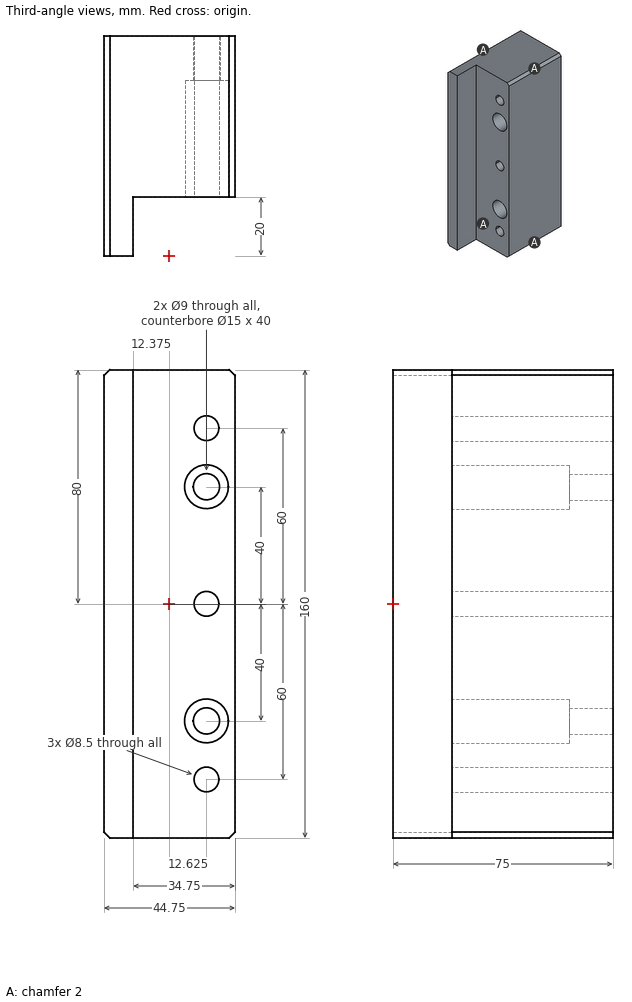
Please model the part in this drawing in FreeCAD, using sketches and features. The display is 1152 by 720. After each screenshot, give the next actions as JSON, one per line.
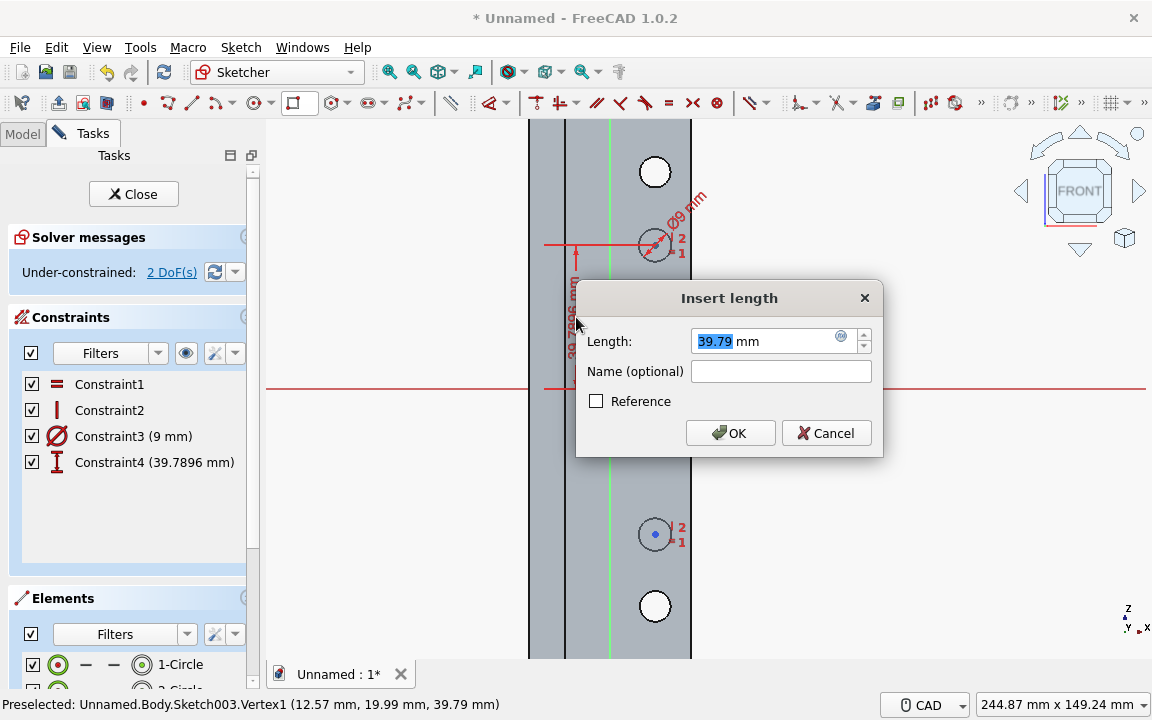
{"action": "type", "text": "40"}
{"action": "key", "text": "Return"}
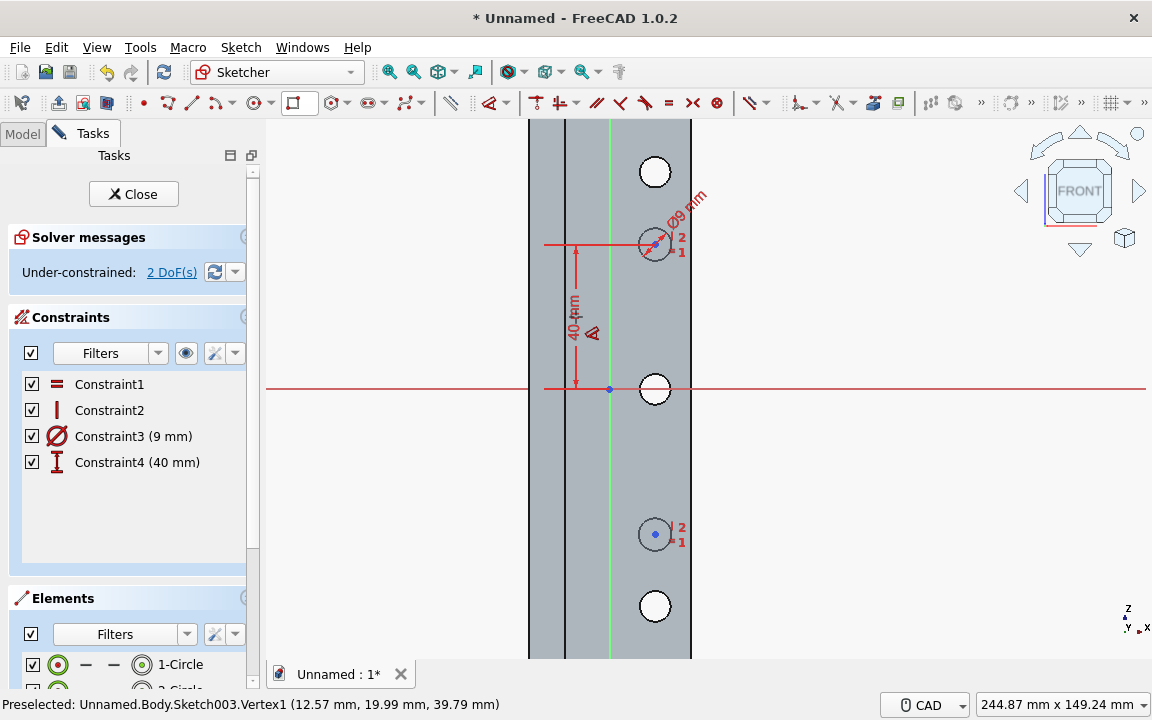
{"action": "left_click", "coordinate": [655, 535]}
{"action": "left_click", "coordinate": [576, 462]}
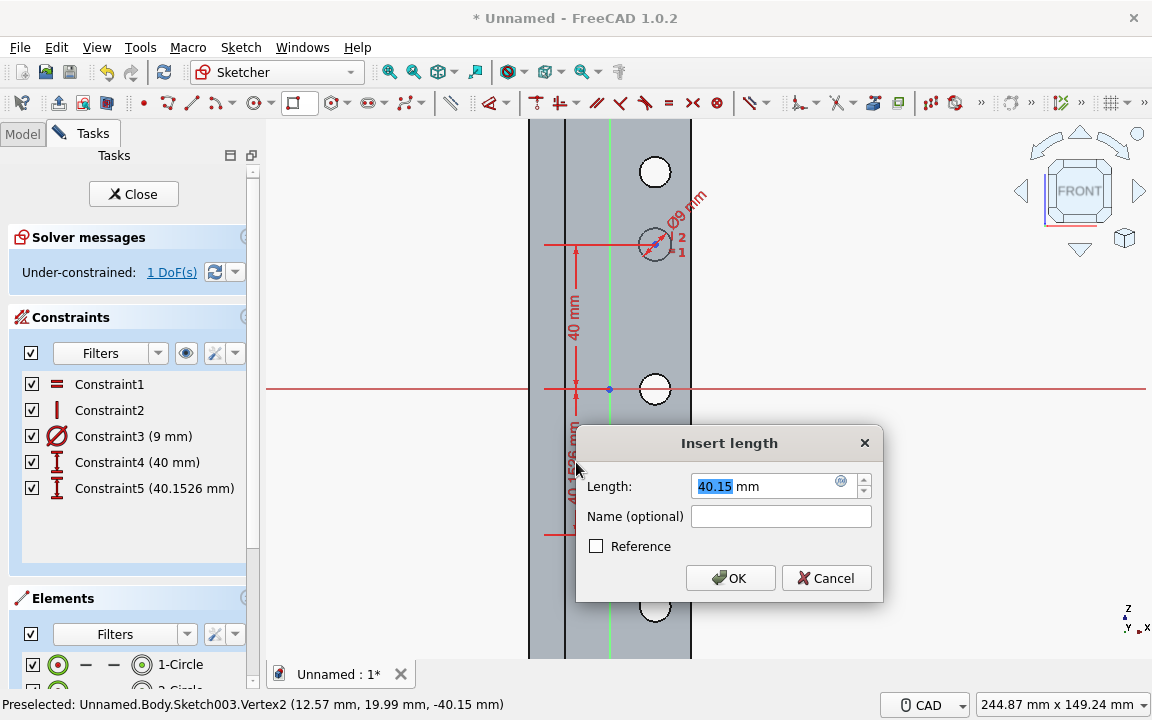
{"action": "type", "text": "40"}
{"action": "key", "text": "Return"}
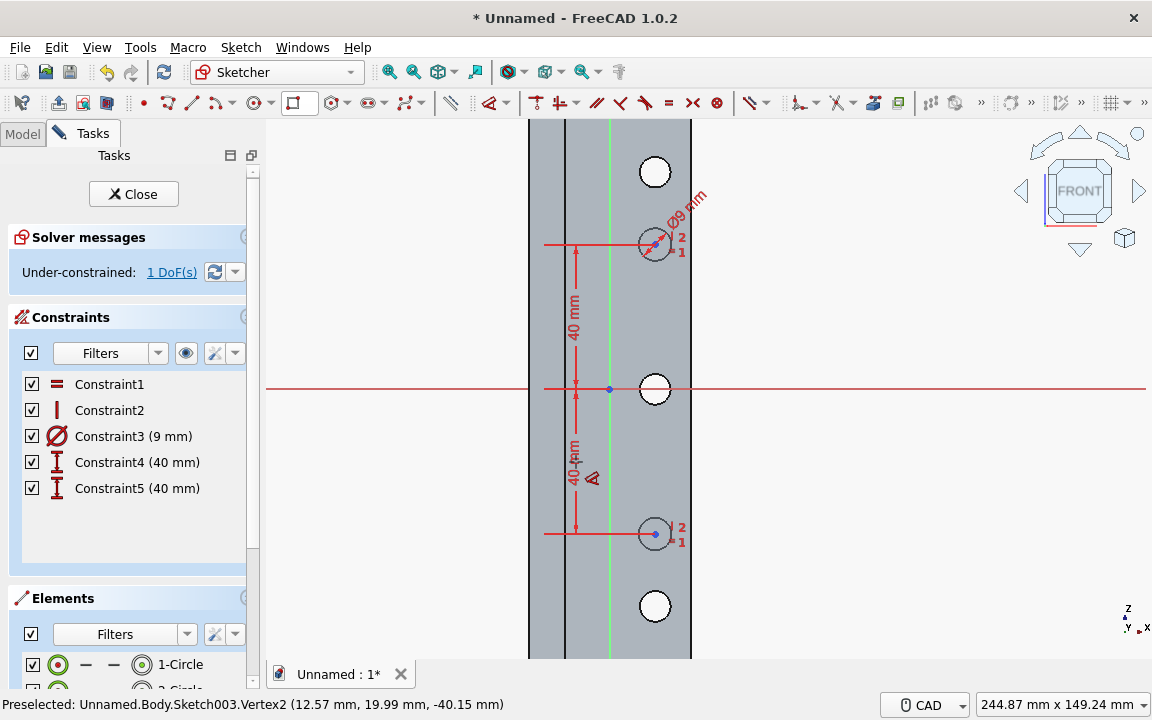
{"action": "left_click", "coordinate": [655, 245]}
{"action": "left_click", "coordinate": [632, 423]}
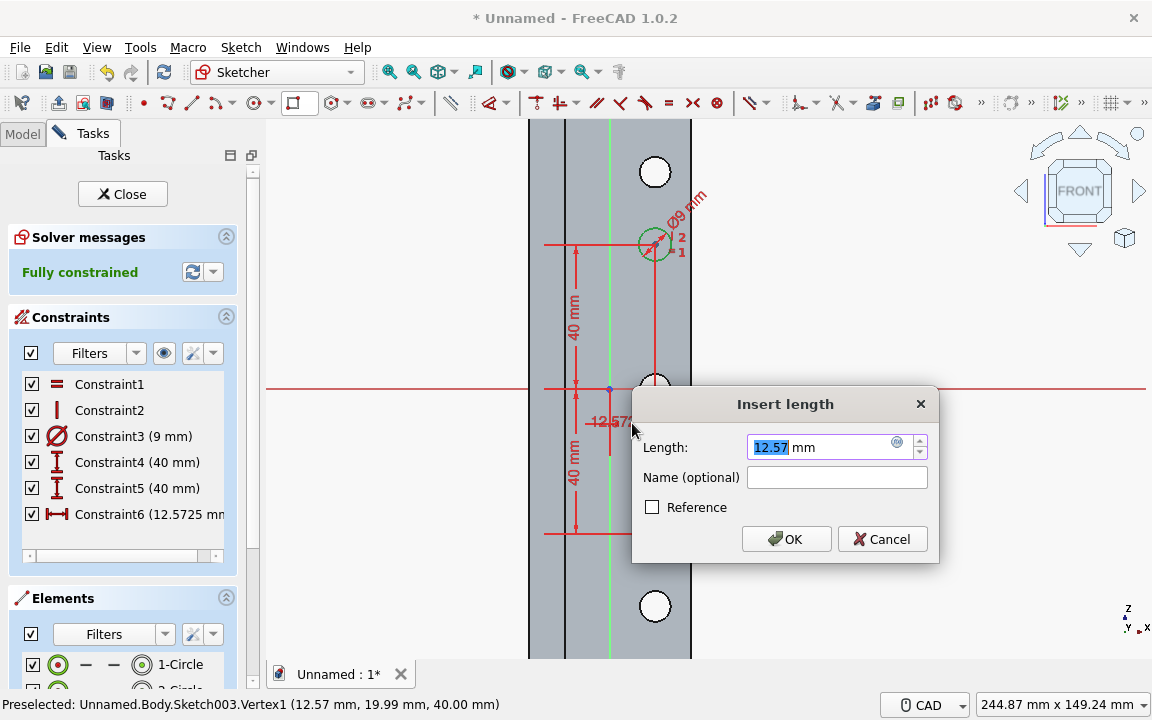
{"action": "type", "text": "12.625"}
{"action": "key", "text": "Return"}
{"action": "key", "text": "Escape"}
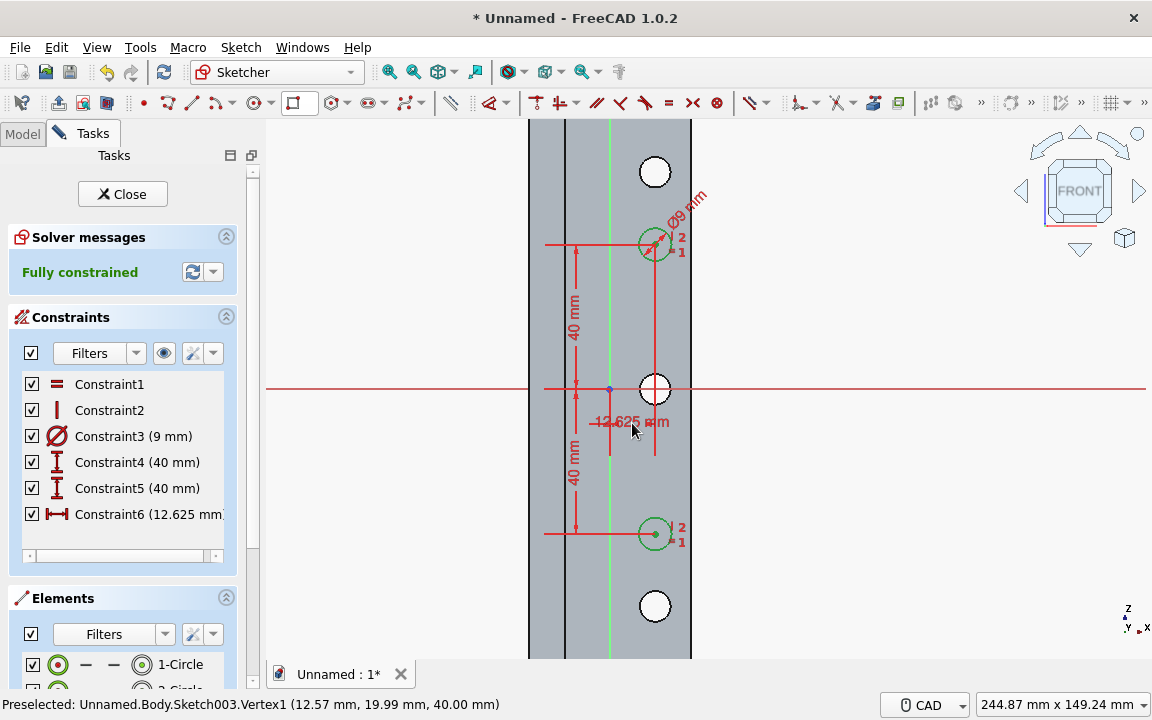
{"action": "left_click", "coordinate": [123, 194]}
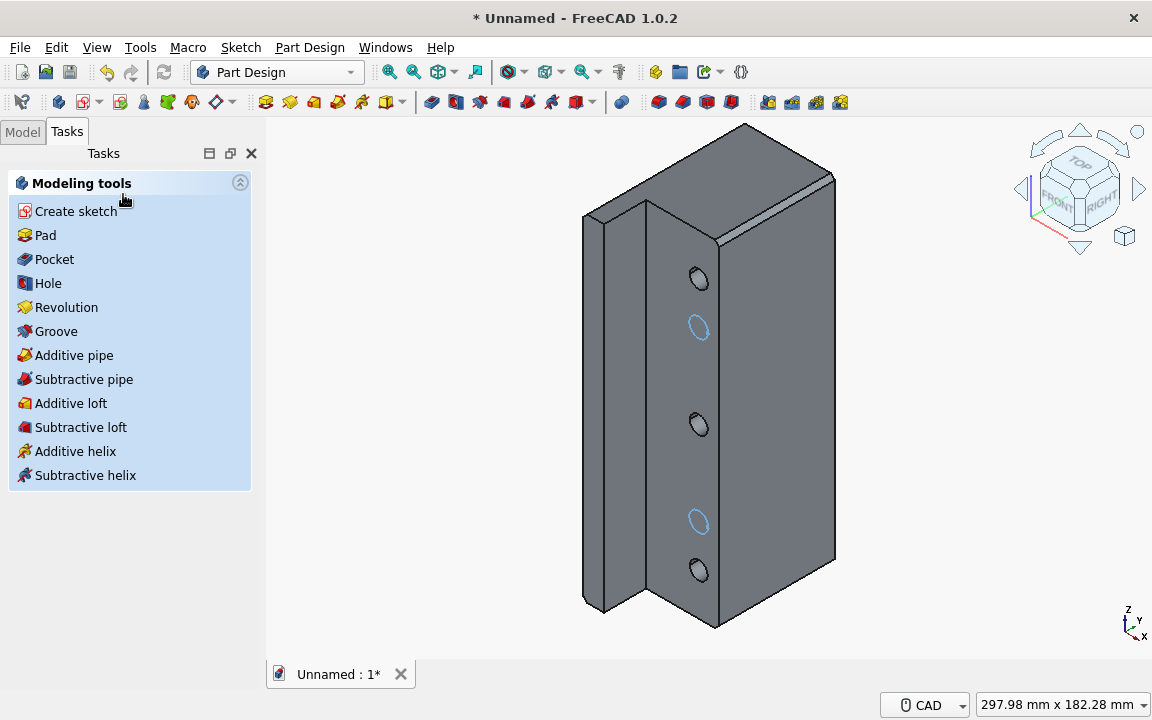
{"action": "left_click", "coordinate": [456, 102]}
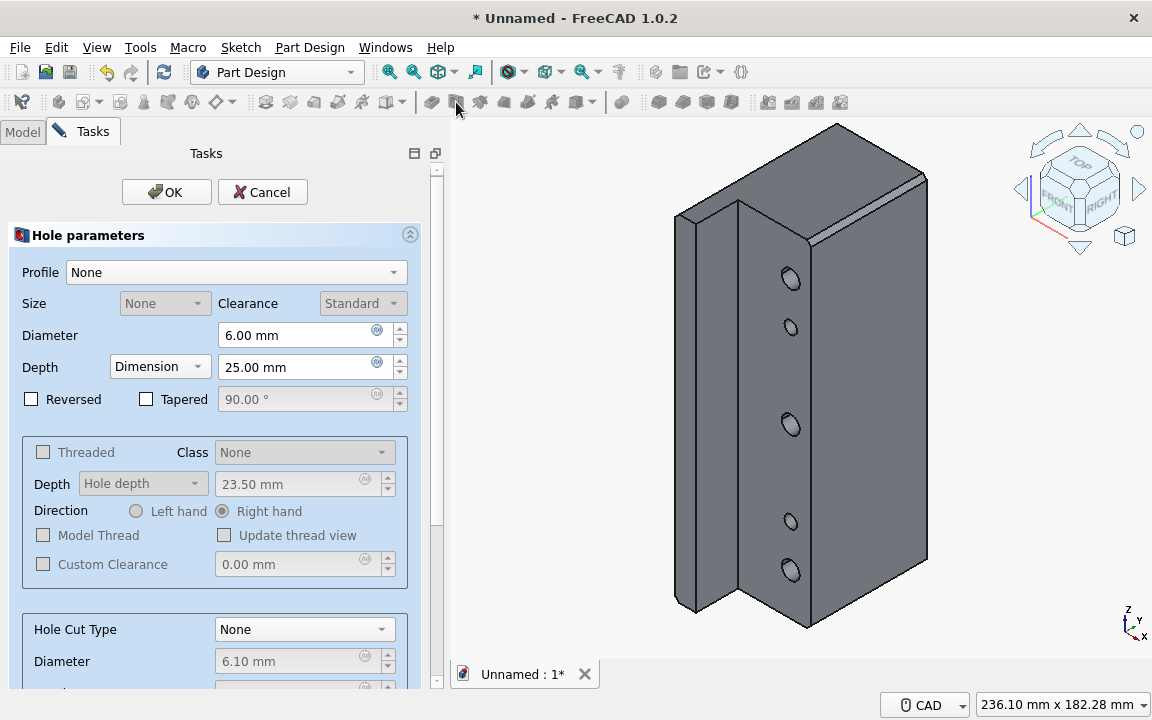
{"action": "triple_click", "coordinate": [305, 335]}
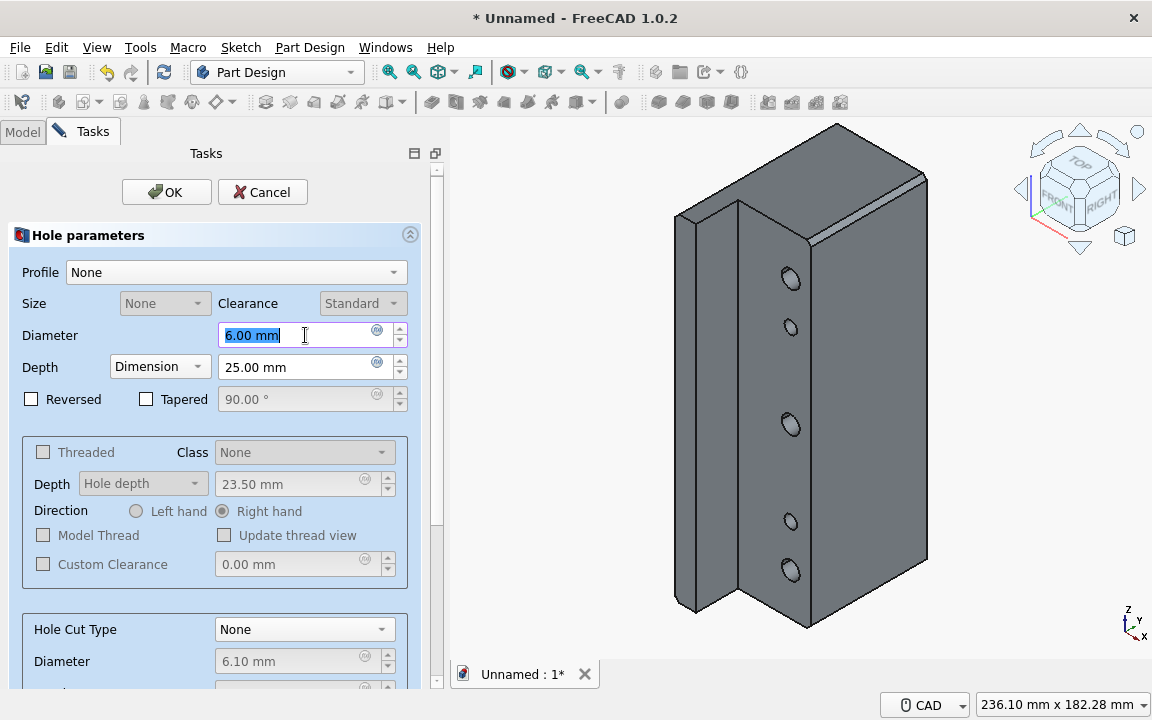
{"action": "type", "text": "9"}
{"action": "key", "text": "Tab"}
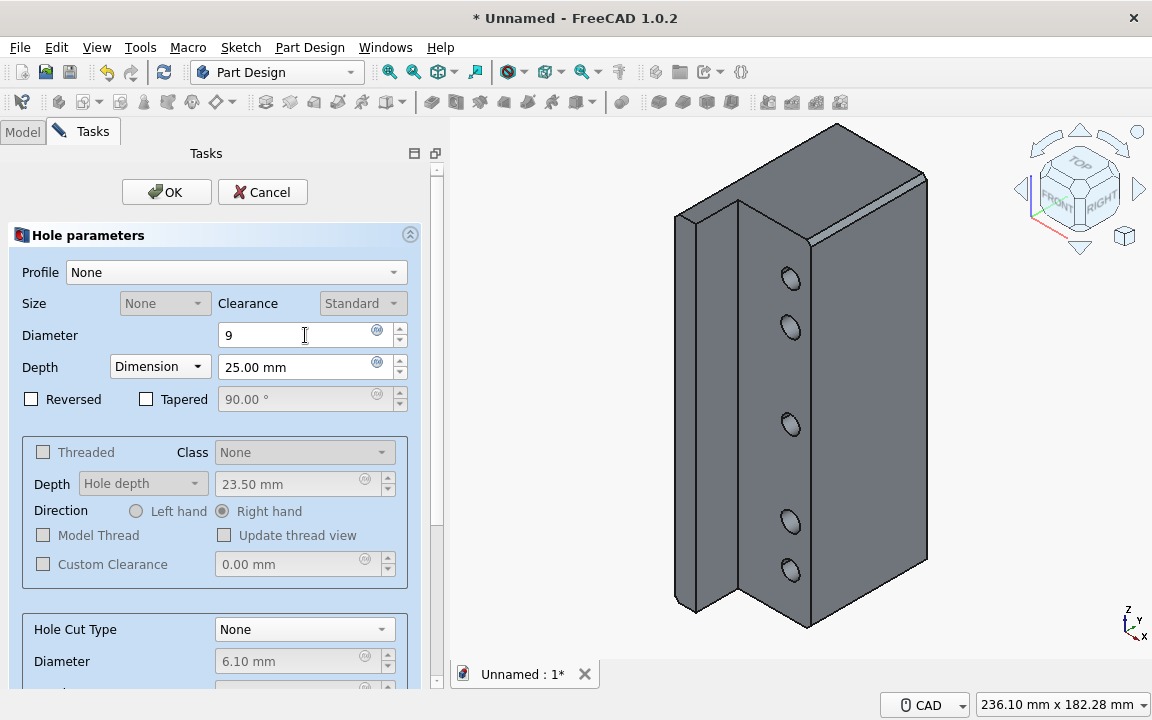
{"action": "left_click", "coordinate": [161, 366]}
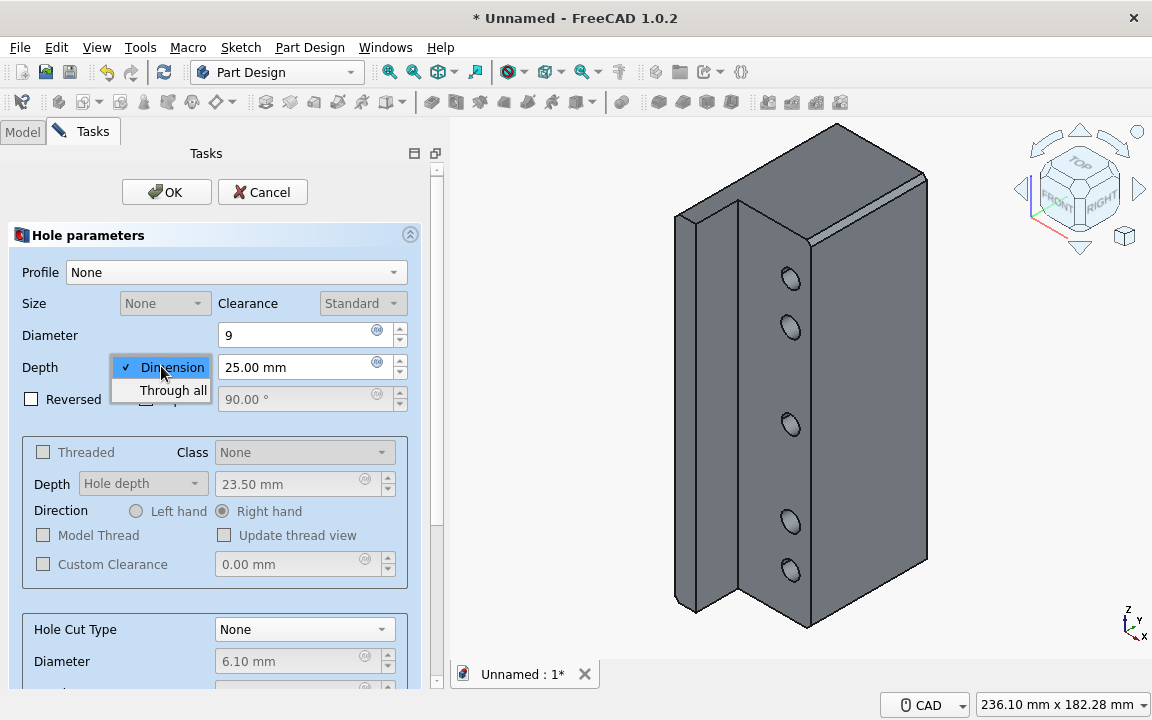
{"action": "left_click", "coordinate": [160, 390]}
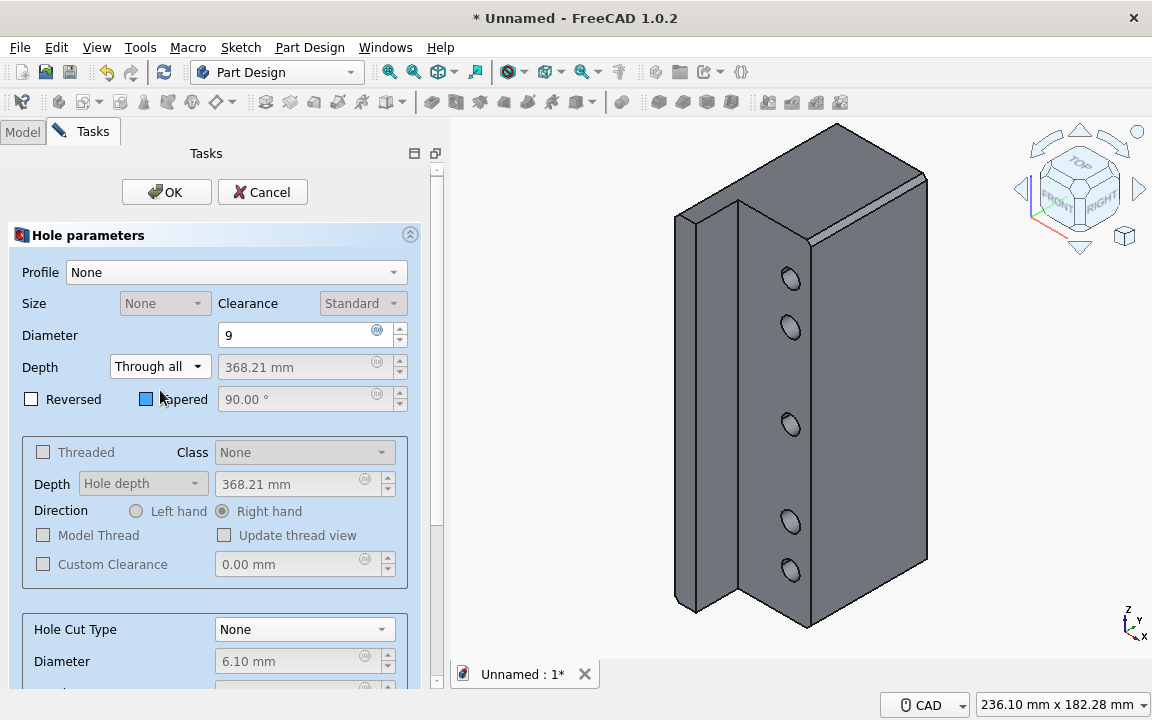
{"action": "left_click", "coordinate": [306, 630]}